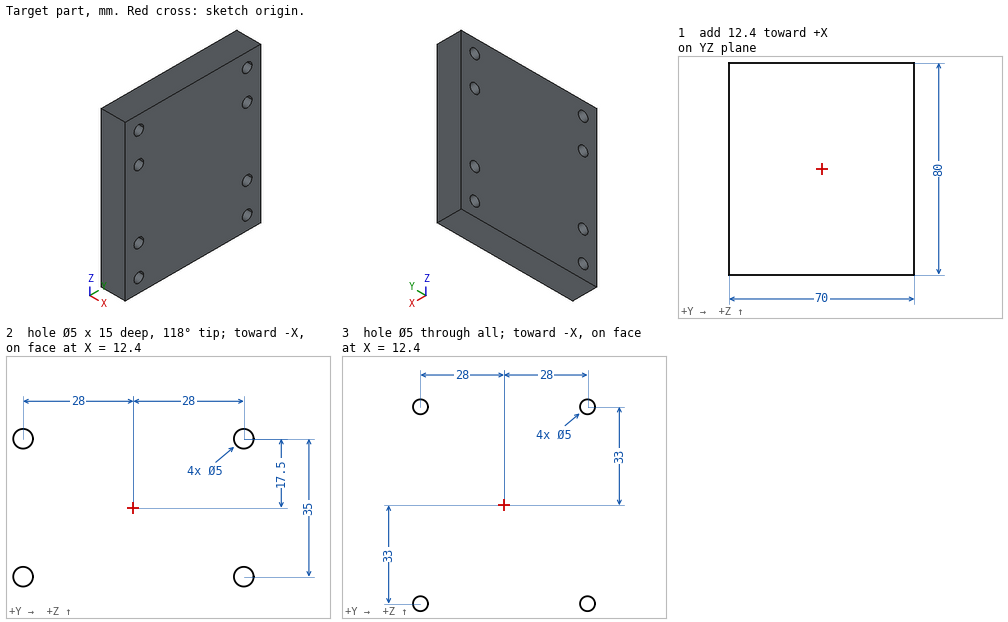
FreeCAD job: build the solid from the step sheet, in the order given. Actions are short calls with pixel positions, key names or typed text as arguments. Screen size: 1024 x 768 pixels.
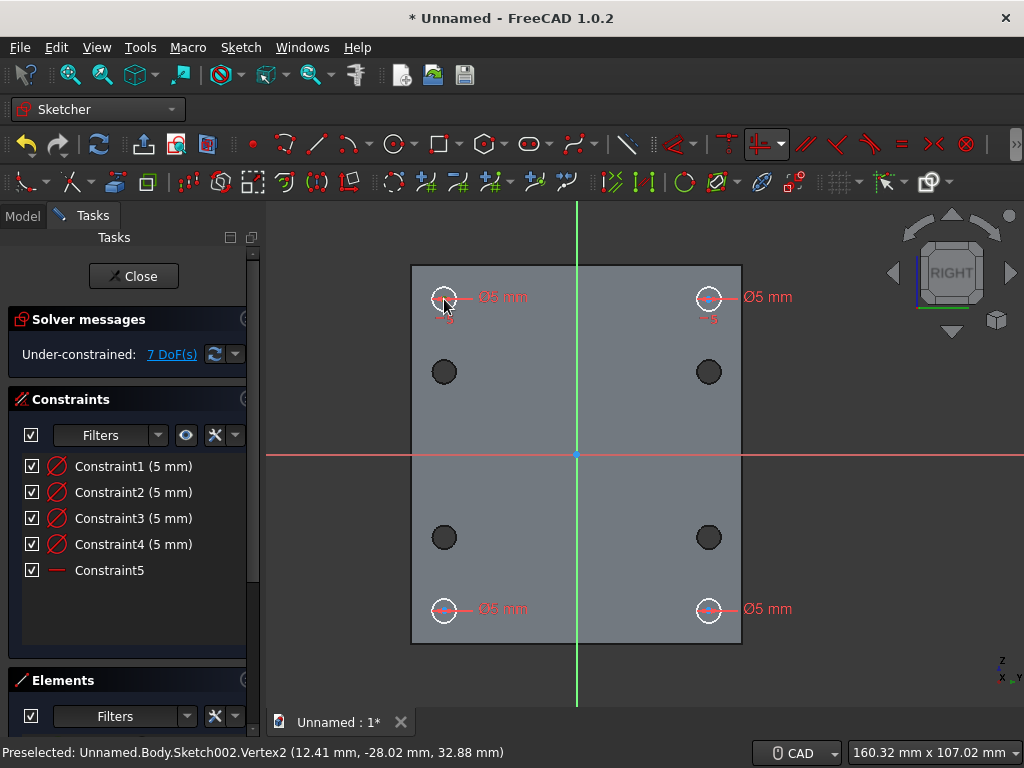
click(444, 611)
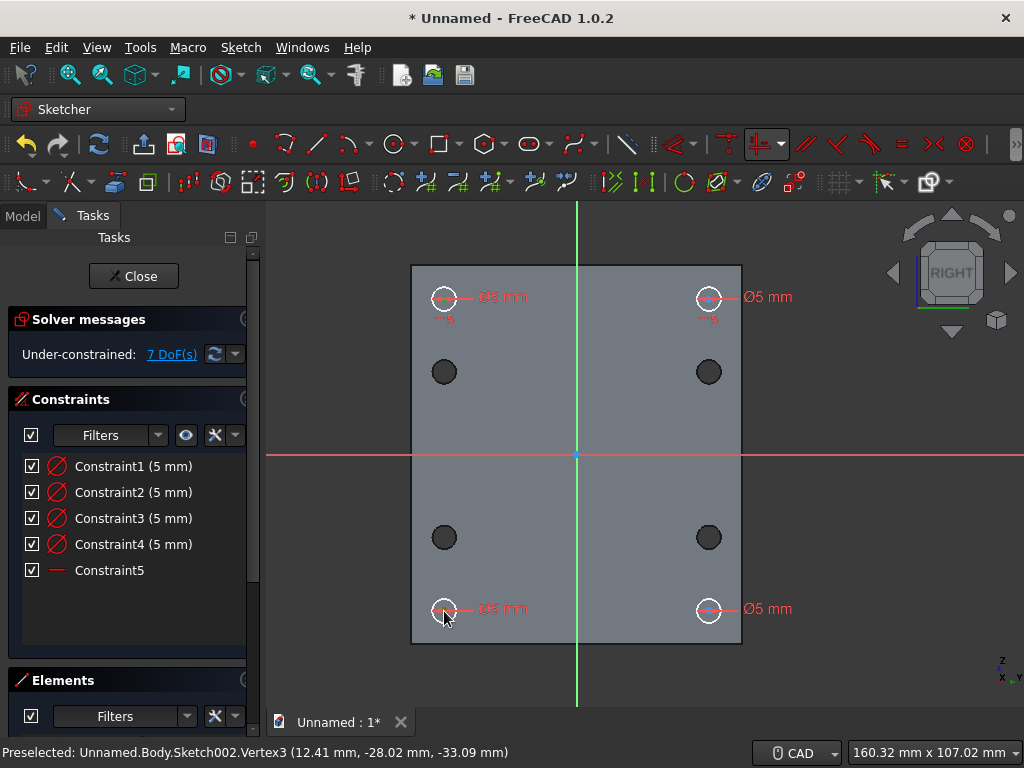
key(v)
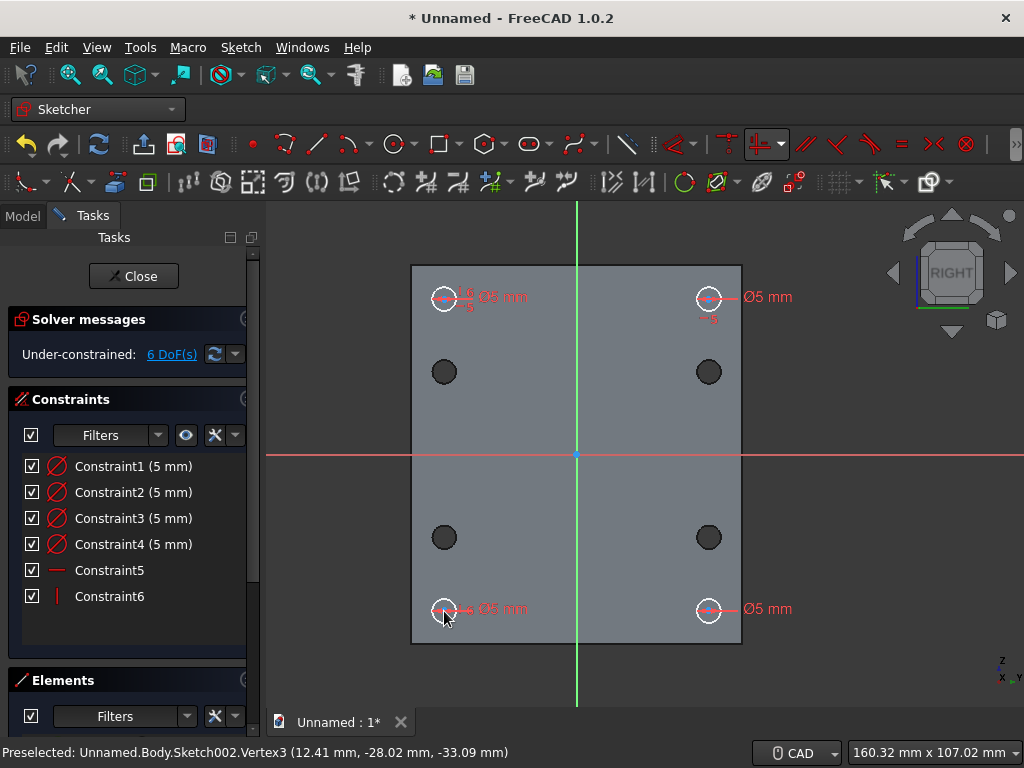
click(709, 299)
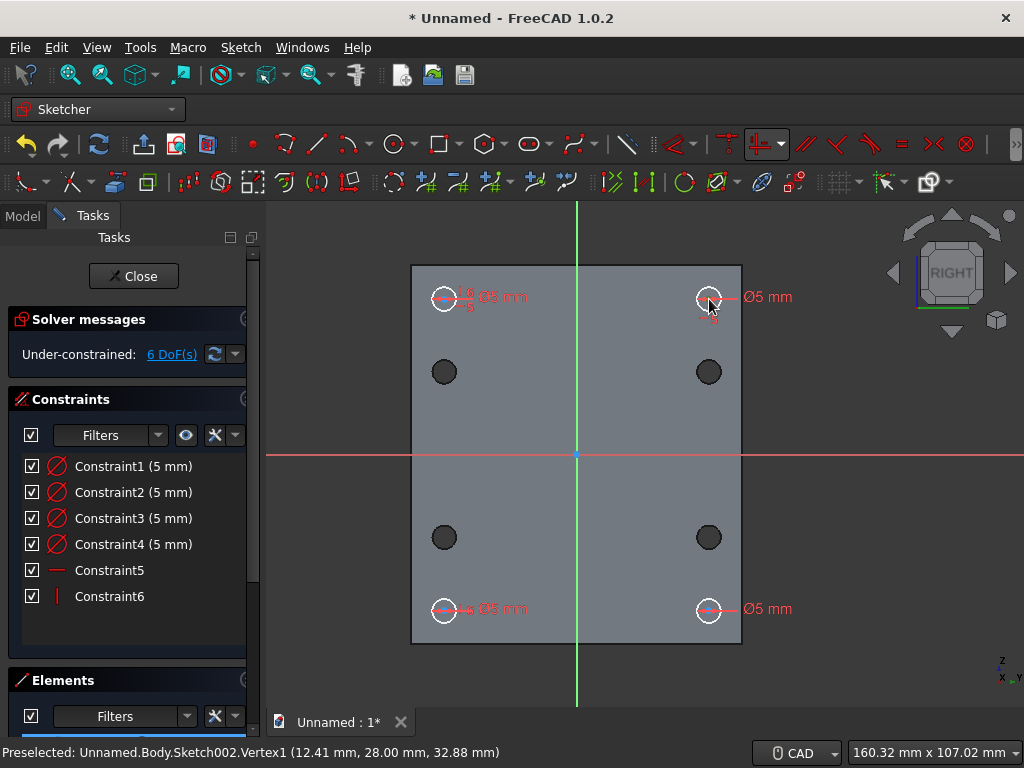
click(709, 611)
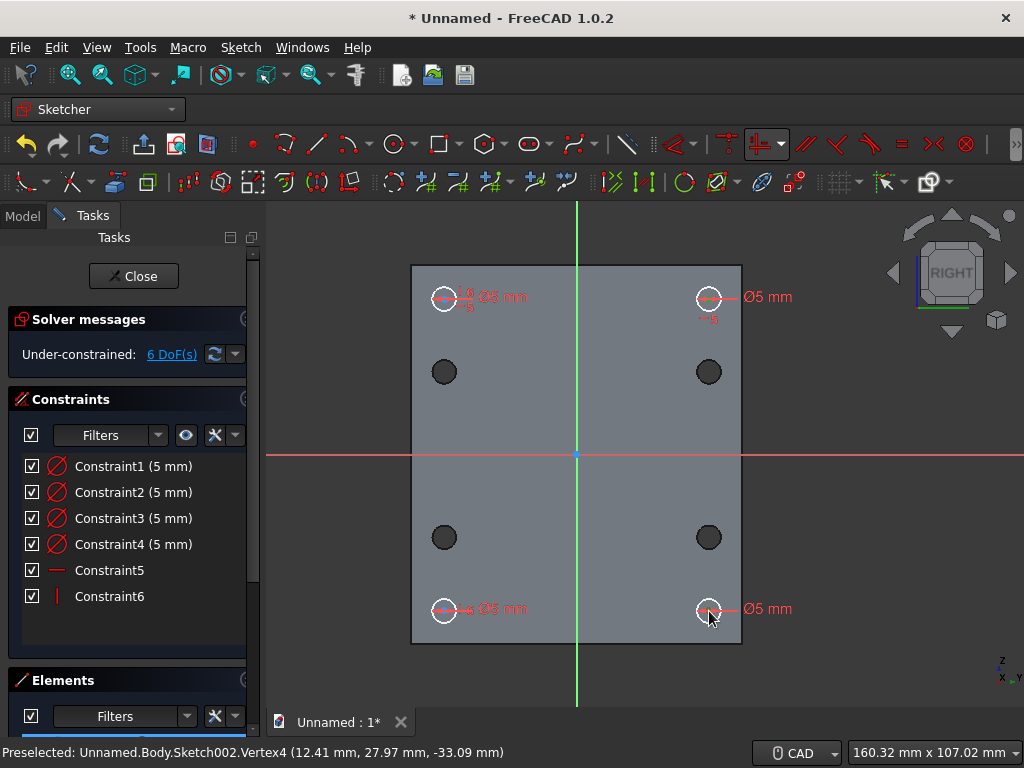
key(v)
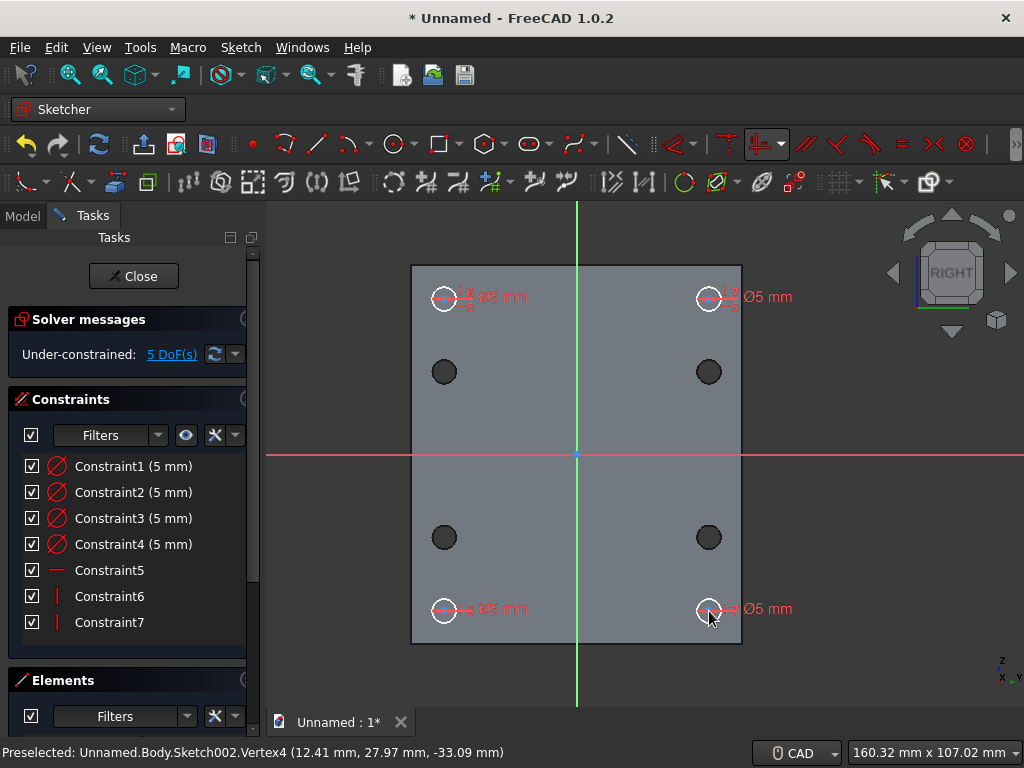
click(444, 611)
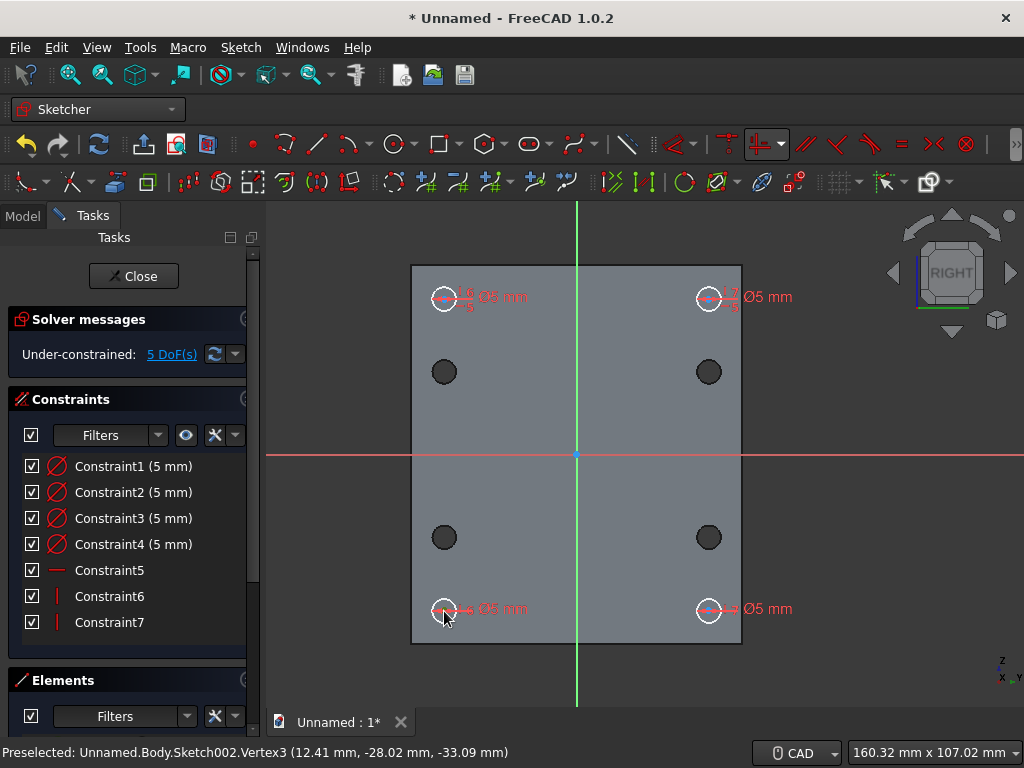
click(709, 611)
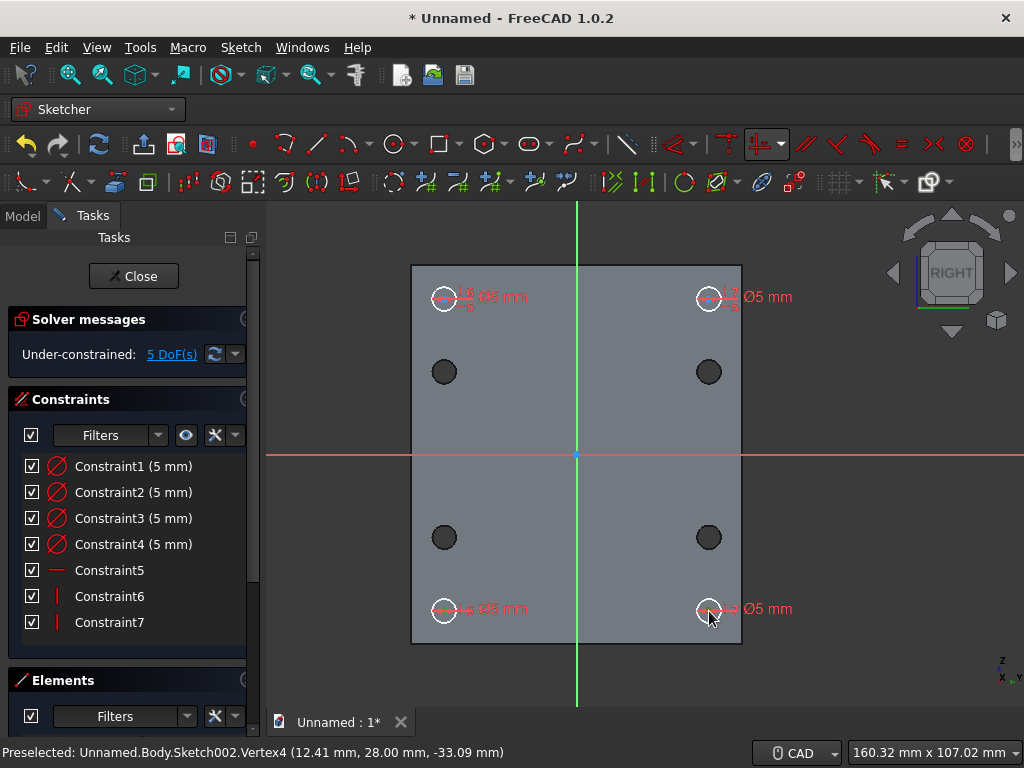
key(h)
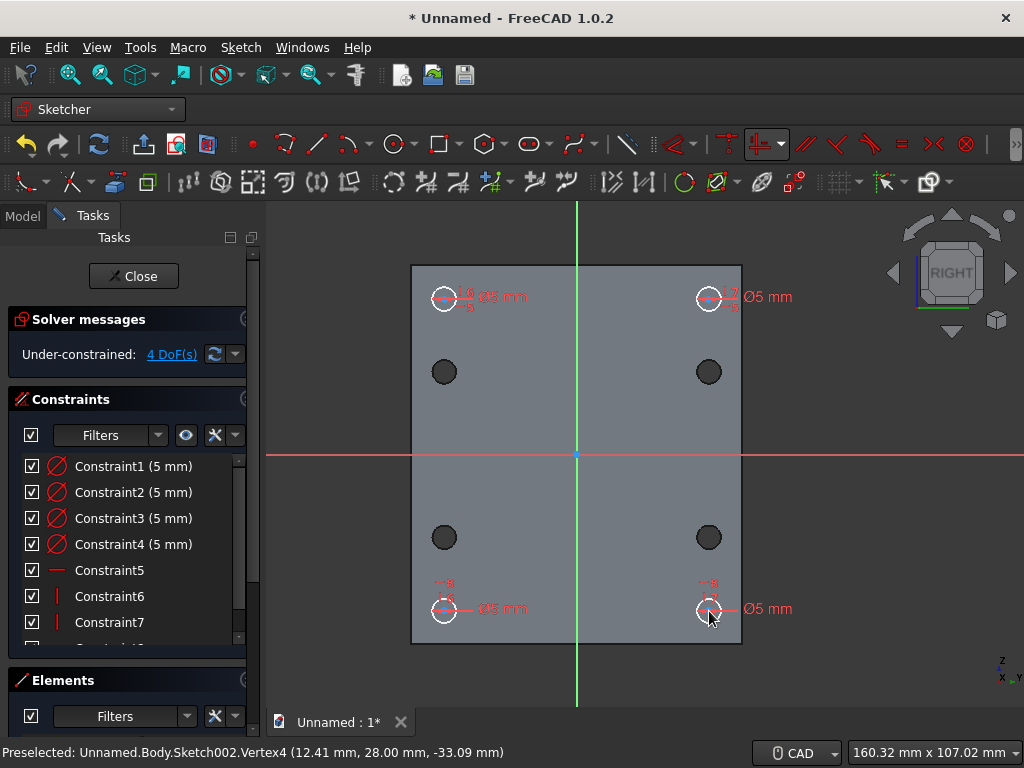
click(709, 299)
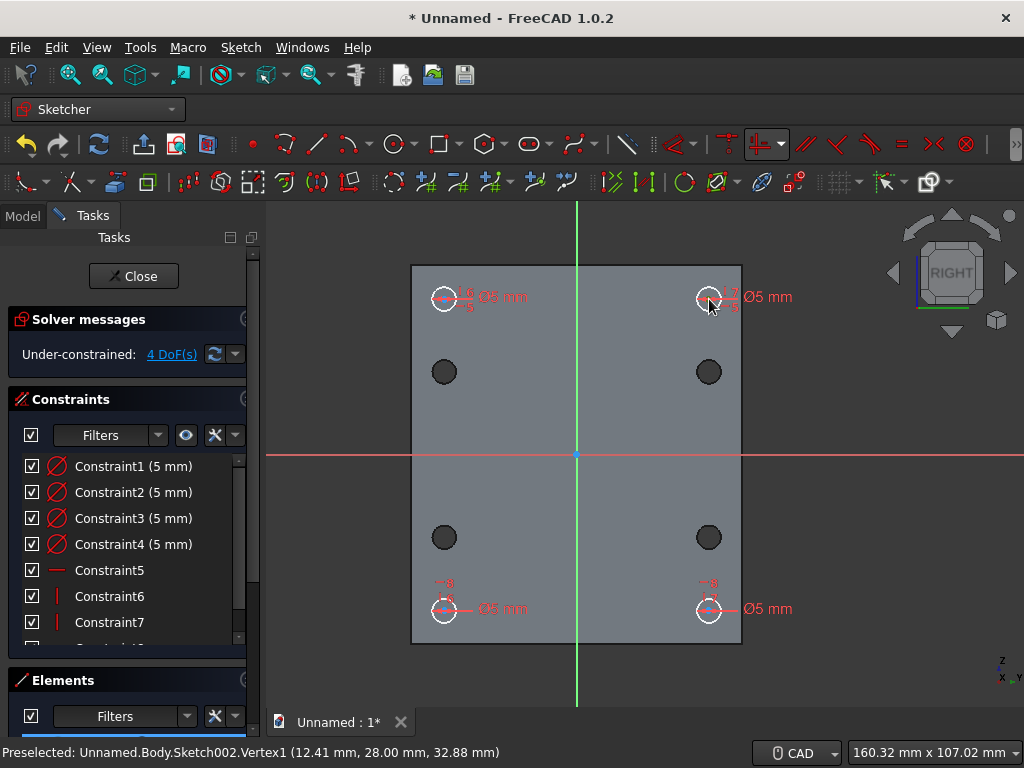
key(l)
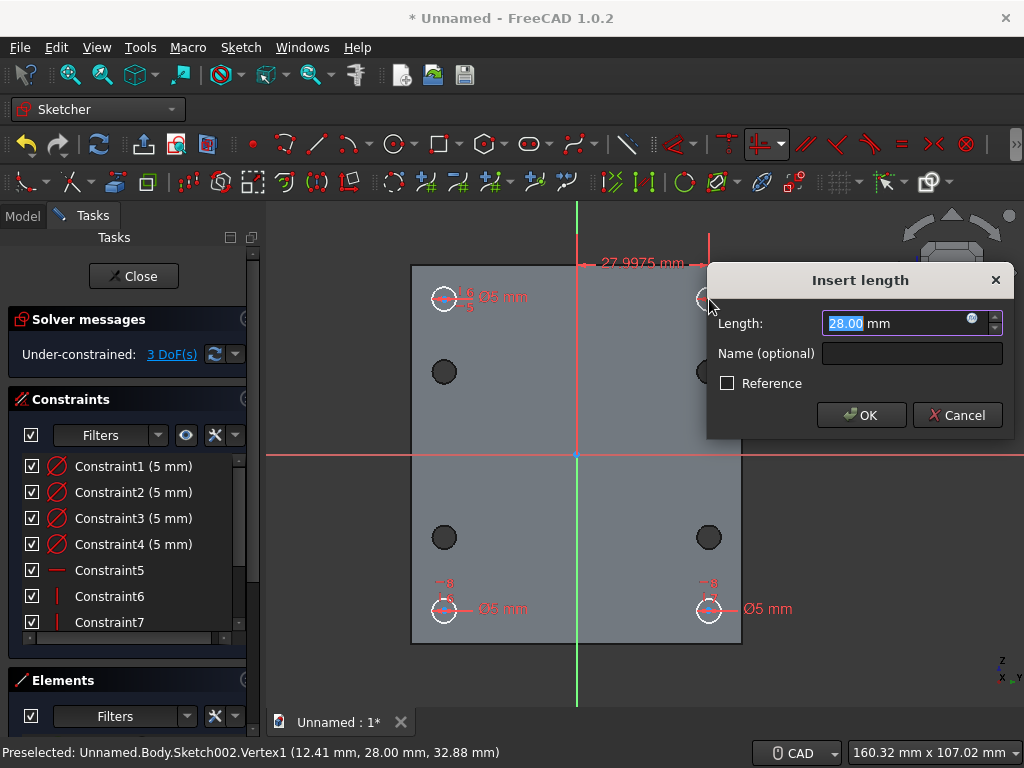
text(28)
key(Return)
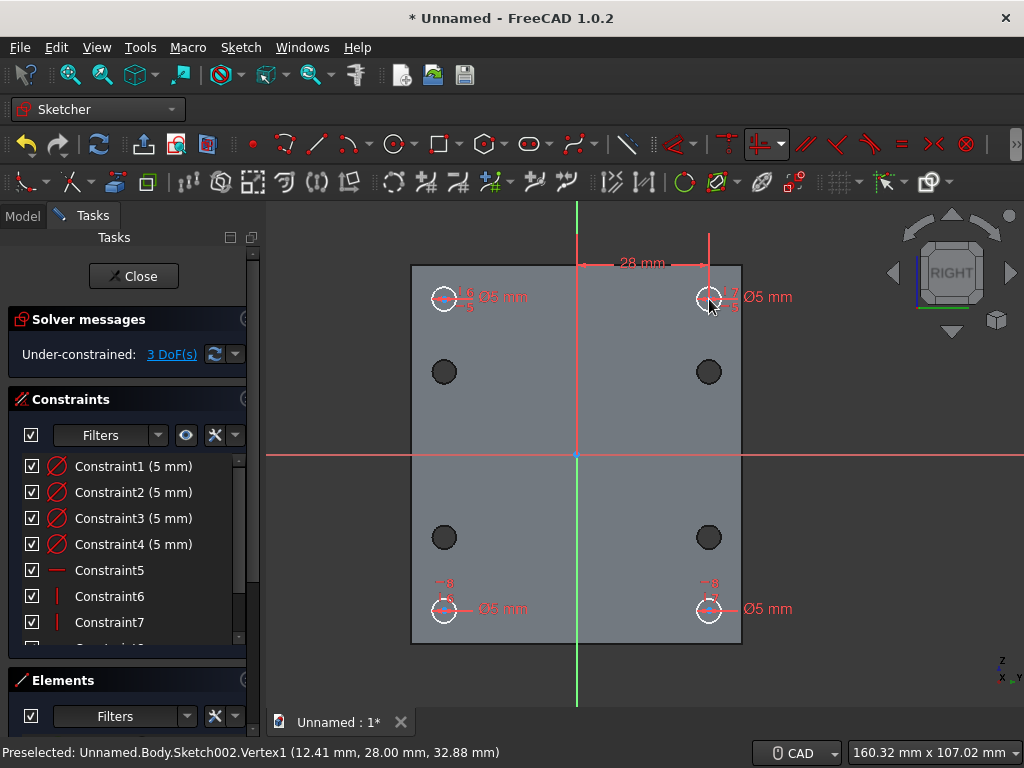
click(709, 299)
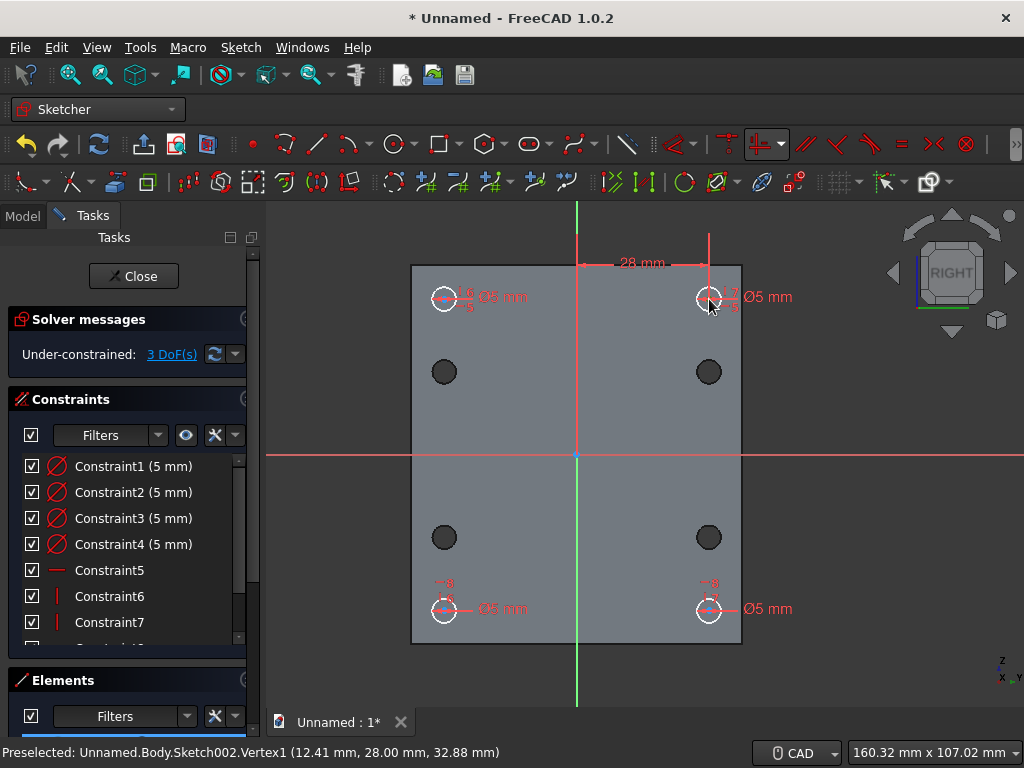
key(i)